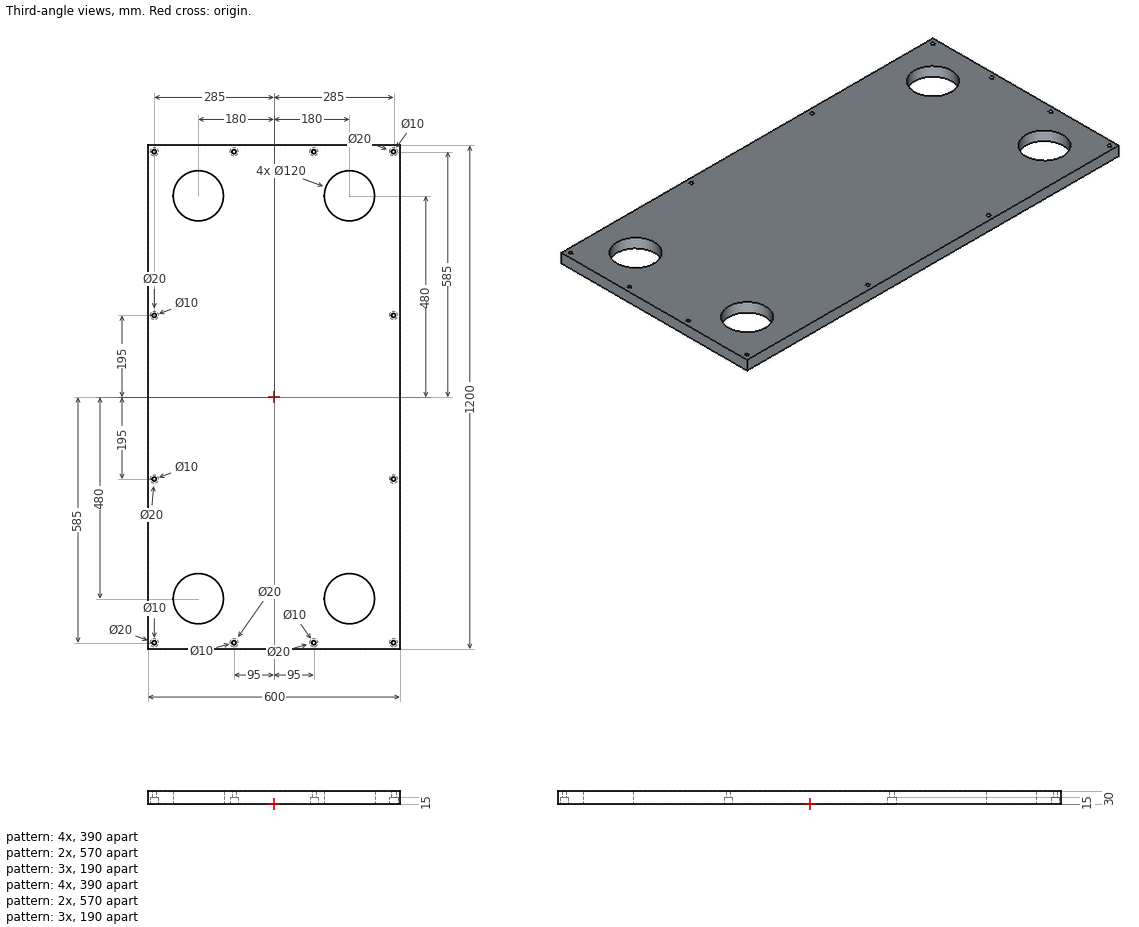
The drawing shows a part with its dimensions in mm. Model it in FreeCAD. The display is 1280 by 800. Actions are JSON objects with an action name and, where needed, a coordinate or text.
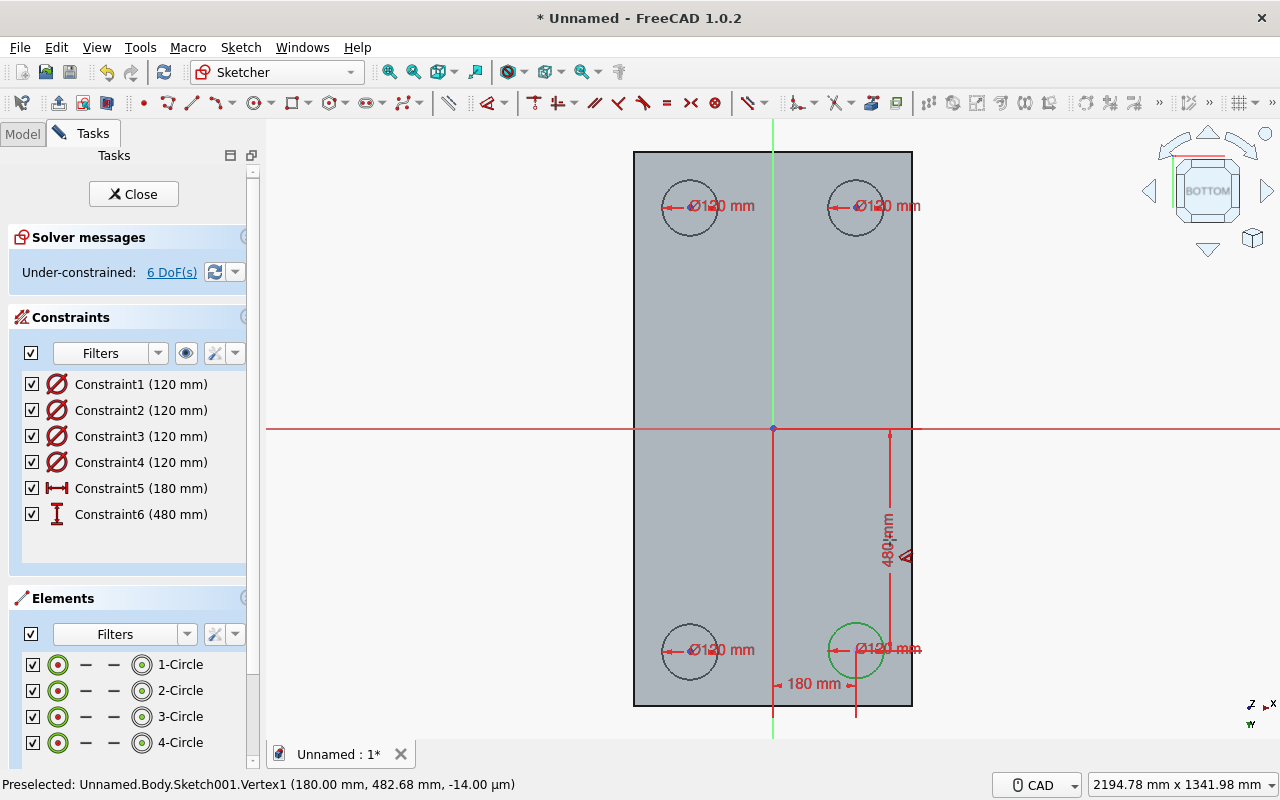
{"action": "left_click", "coordinate": [690, 652]}
{"action": "left_click", "coordinate": [732, 686]}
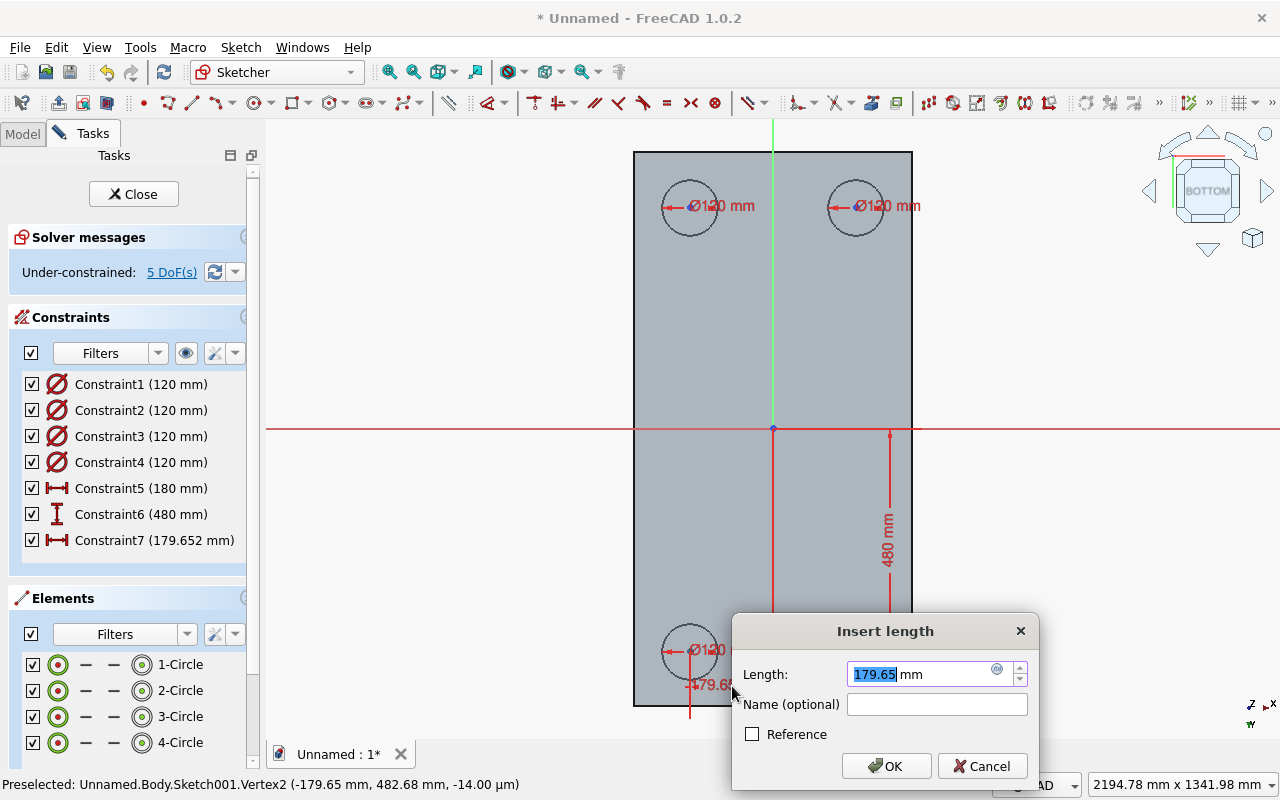
{"action": "type", "text": "180"}
{"action": "key", "text": "Return"}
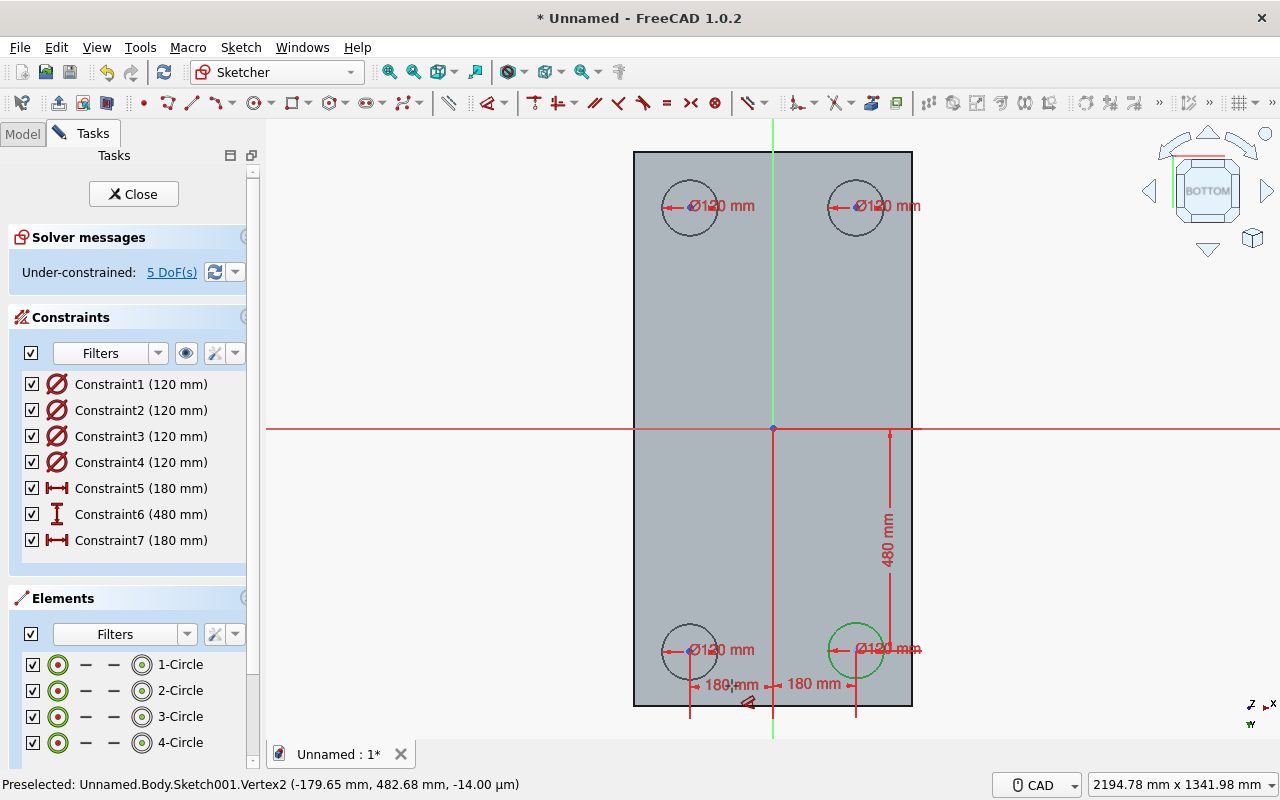
{"action": "left_click", "coordinate": [690, 652]}
{"action": "left_click", "coordinate": [656, 540]}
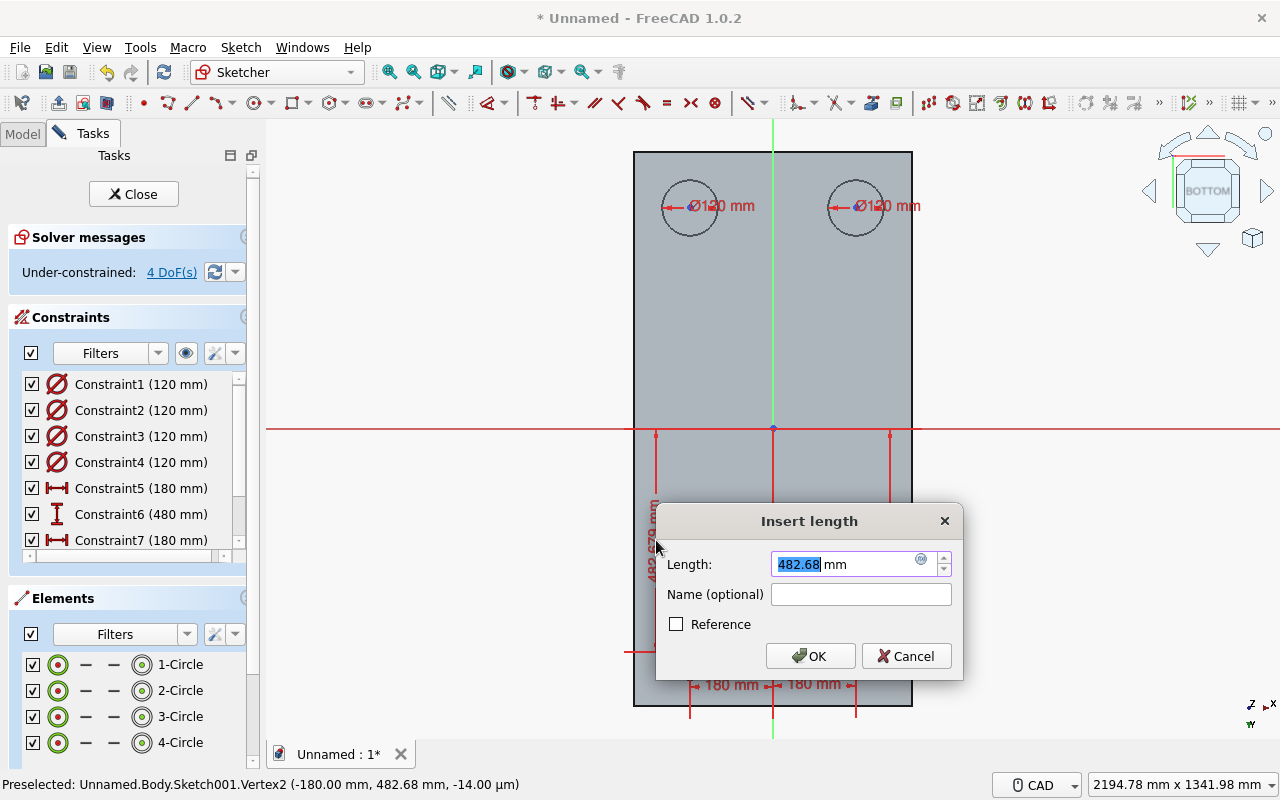
{"action": "type", "text": "480"}
{"action": "key", "text": "Return"}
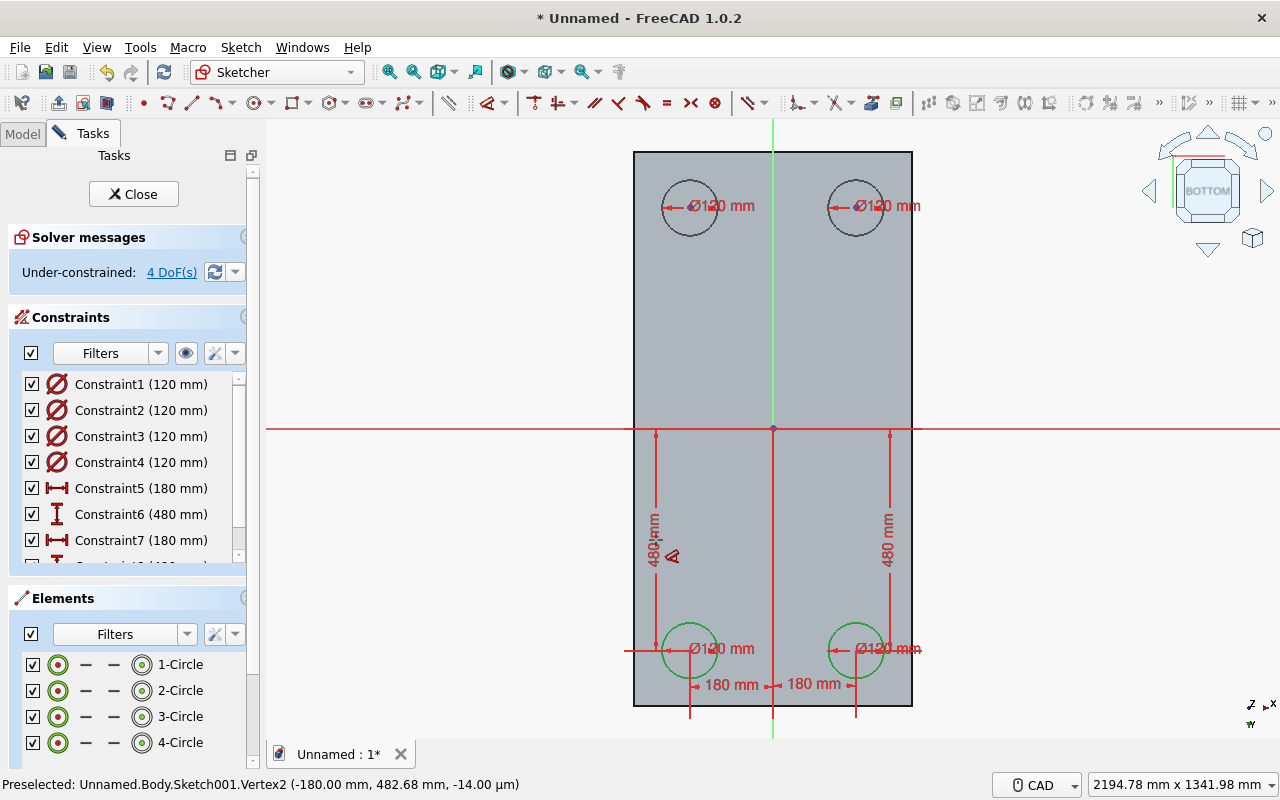
{"action": "left_click", "coordinate": [690, 208]}
{"action": "left_click", "coordinate": [732, 174]}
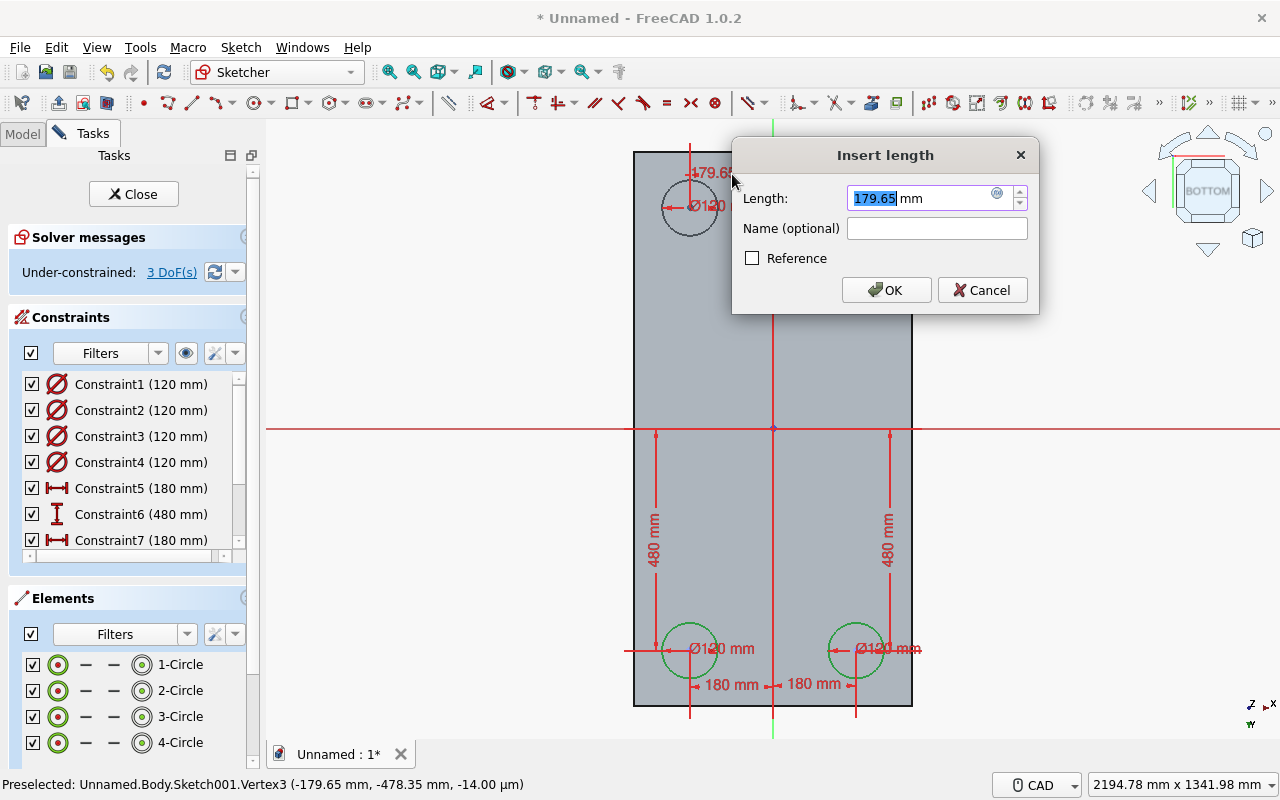
{"action": "type", "text": "180"}
{"action": "key", "text": "Return"}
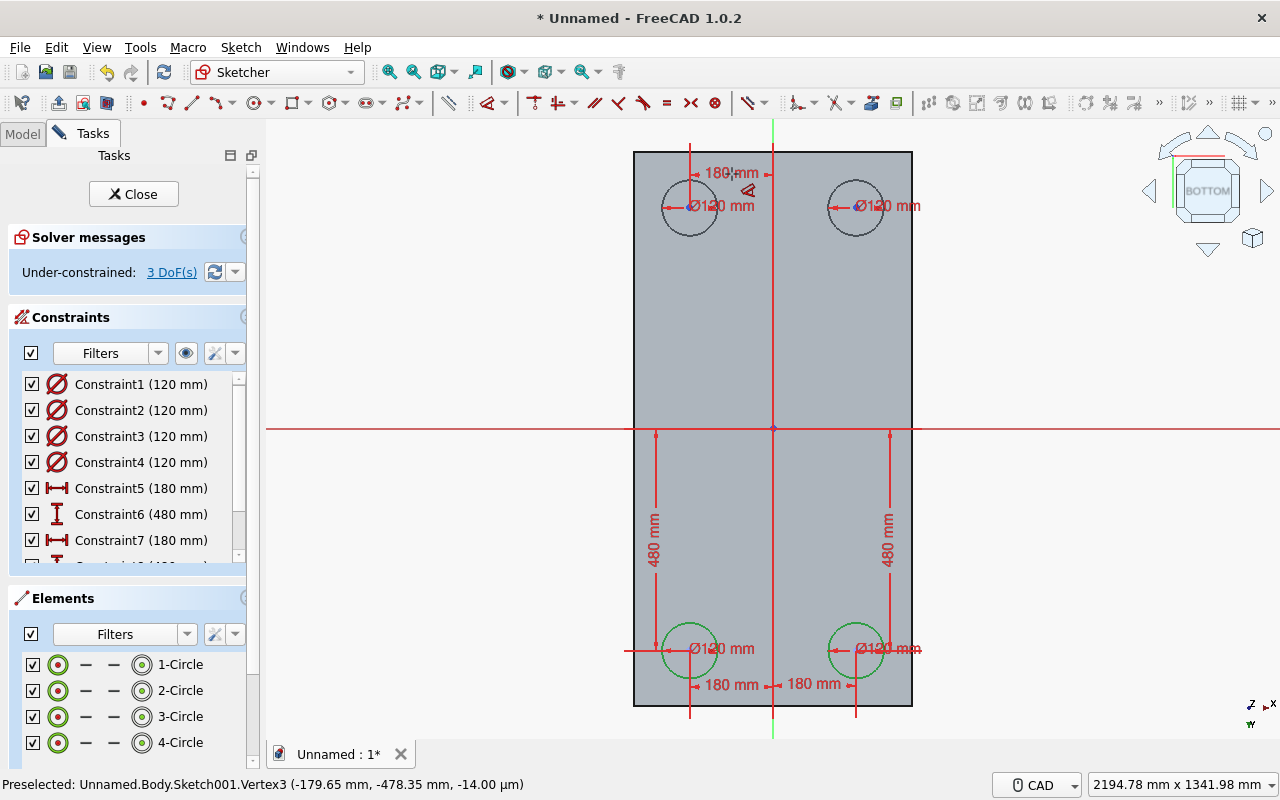
{"action": "left_click", "coordinate": [690, 208]}
{"action": "left_click", "coordinate": [656, 318]}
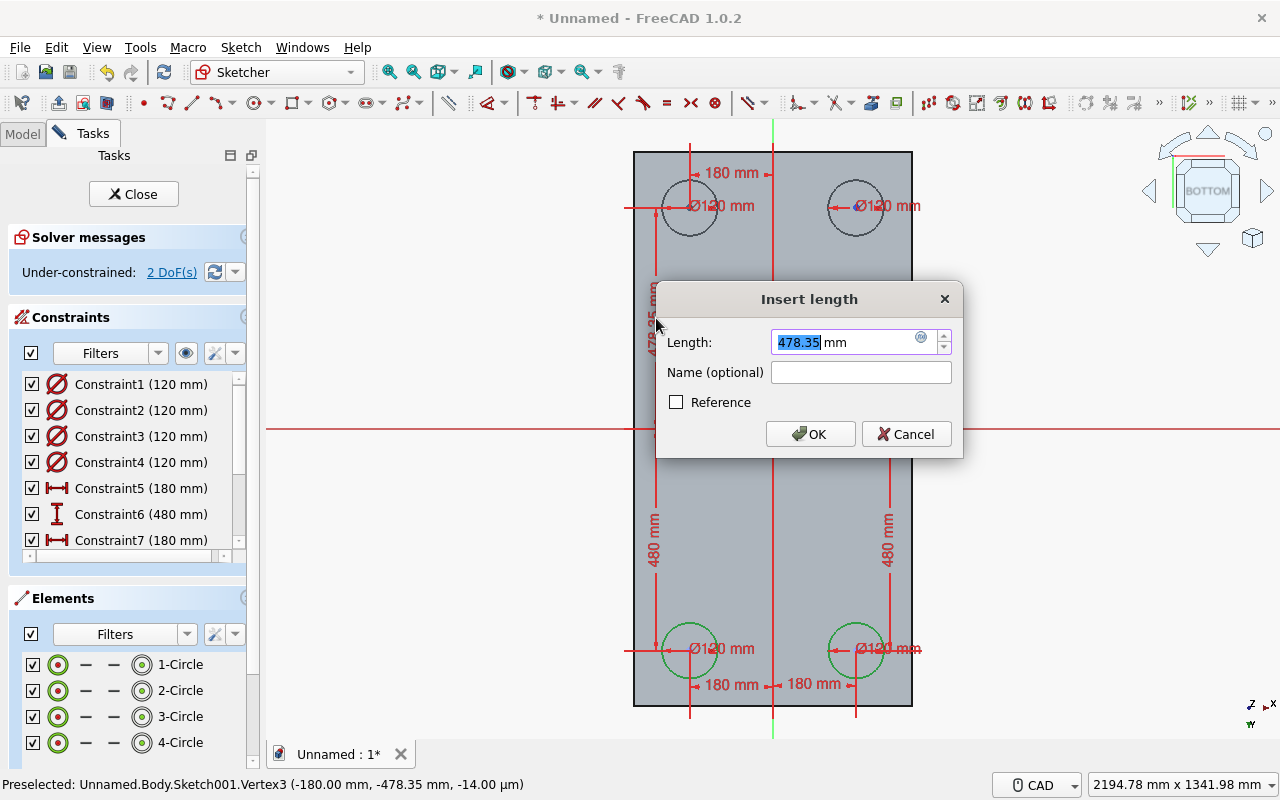
{"action": "type", "text": "480"}
{"action": "key", "text": "Return"}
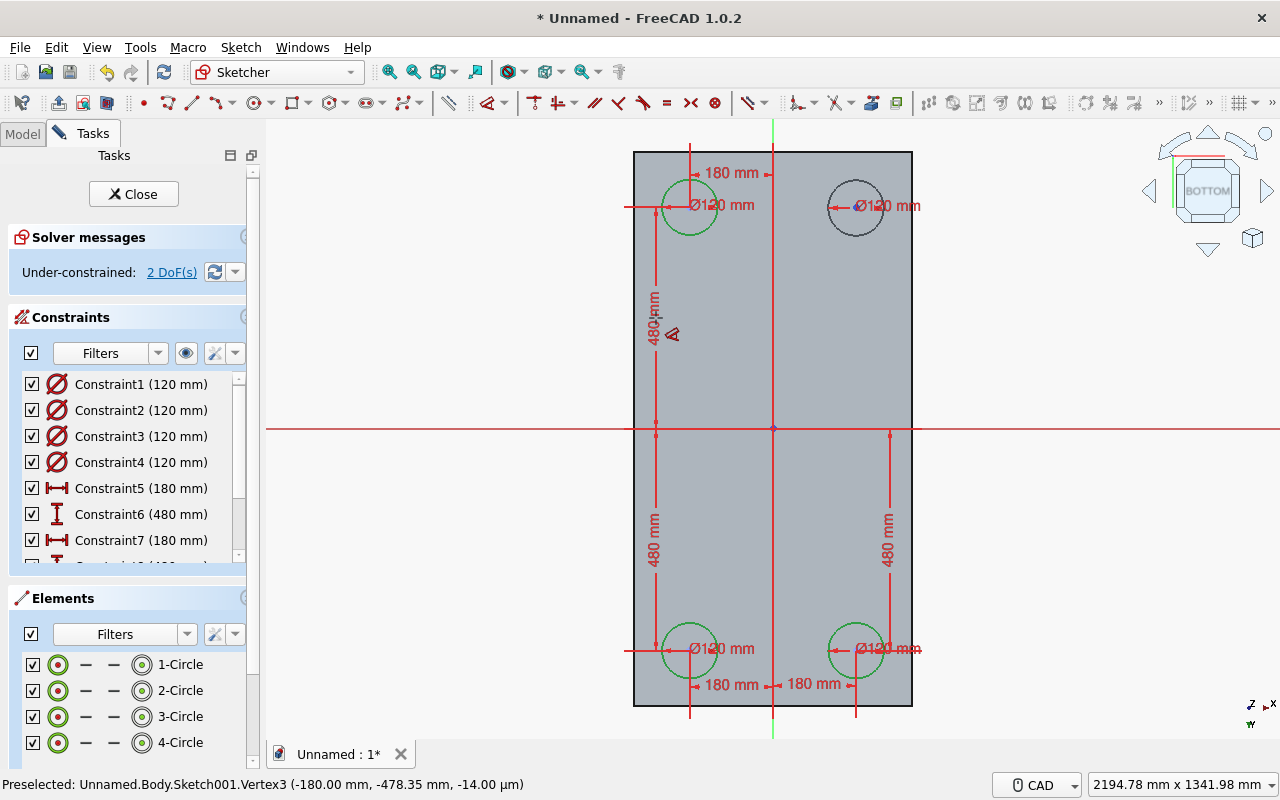
{"action": "left_click", "coordinate": [856, 208]}
{"action": "left_click", "coordinate": [814, 174]}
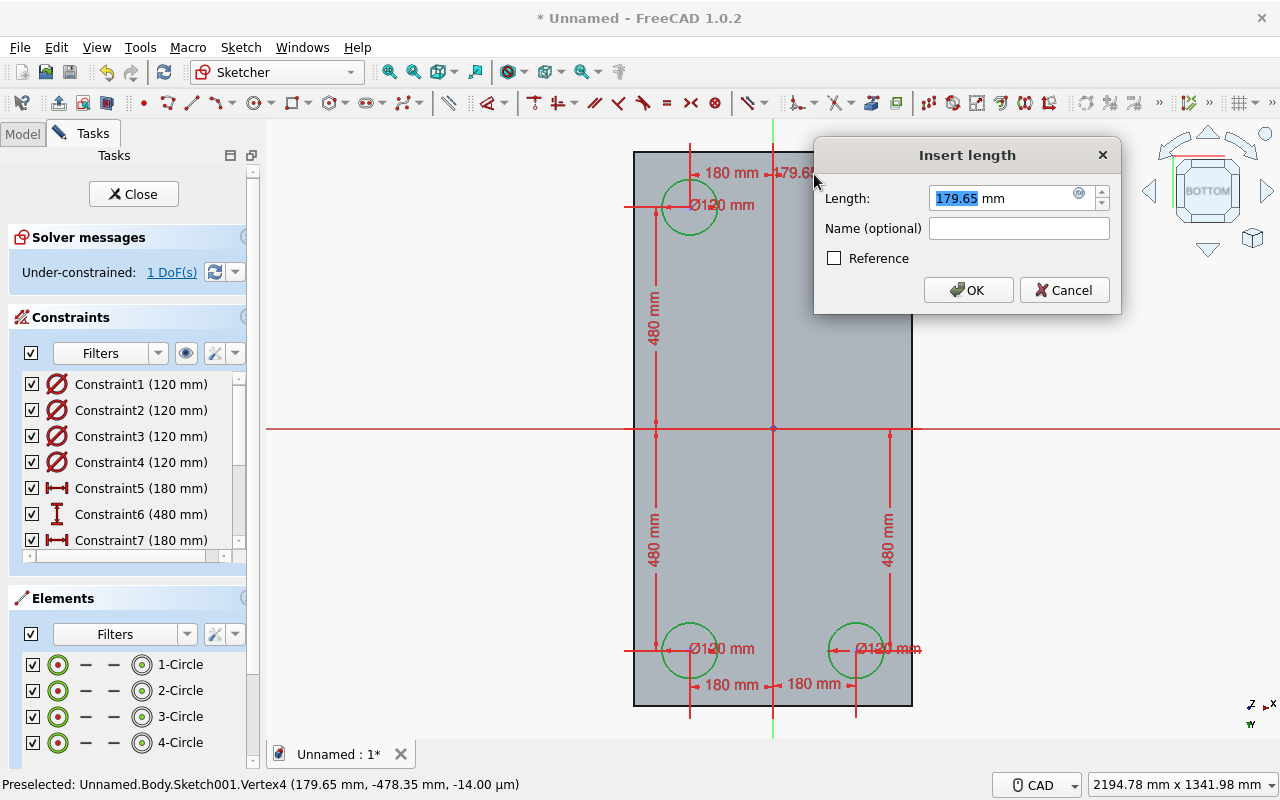
{"action": "type", "text": "180"}
{"action": "key", "text": "Return"}